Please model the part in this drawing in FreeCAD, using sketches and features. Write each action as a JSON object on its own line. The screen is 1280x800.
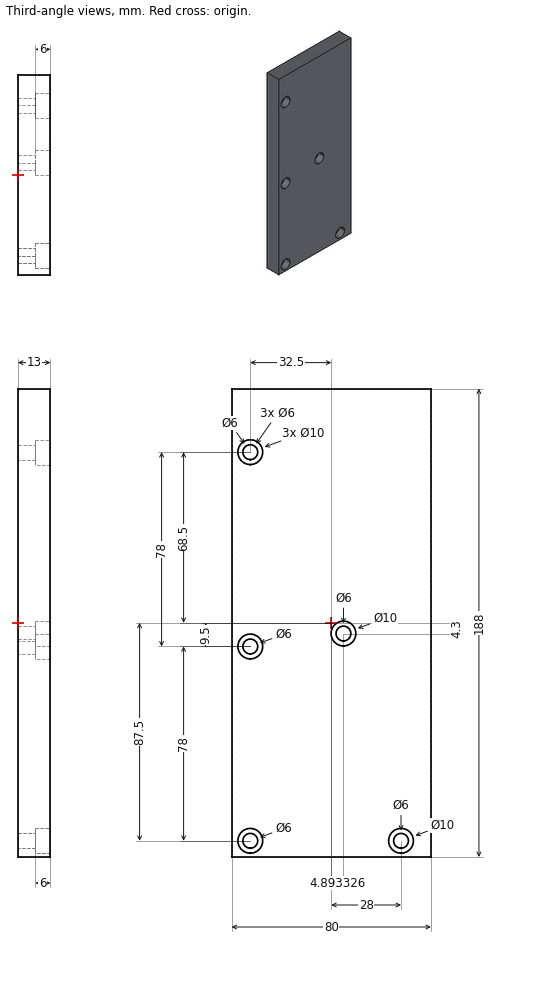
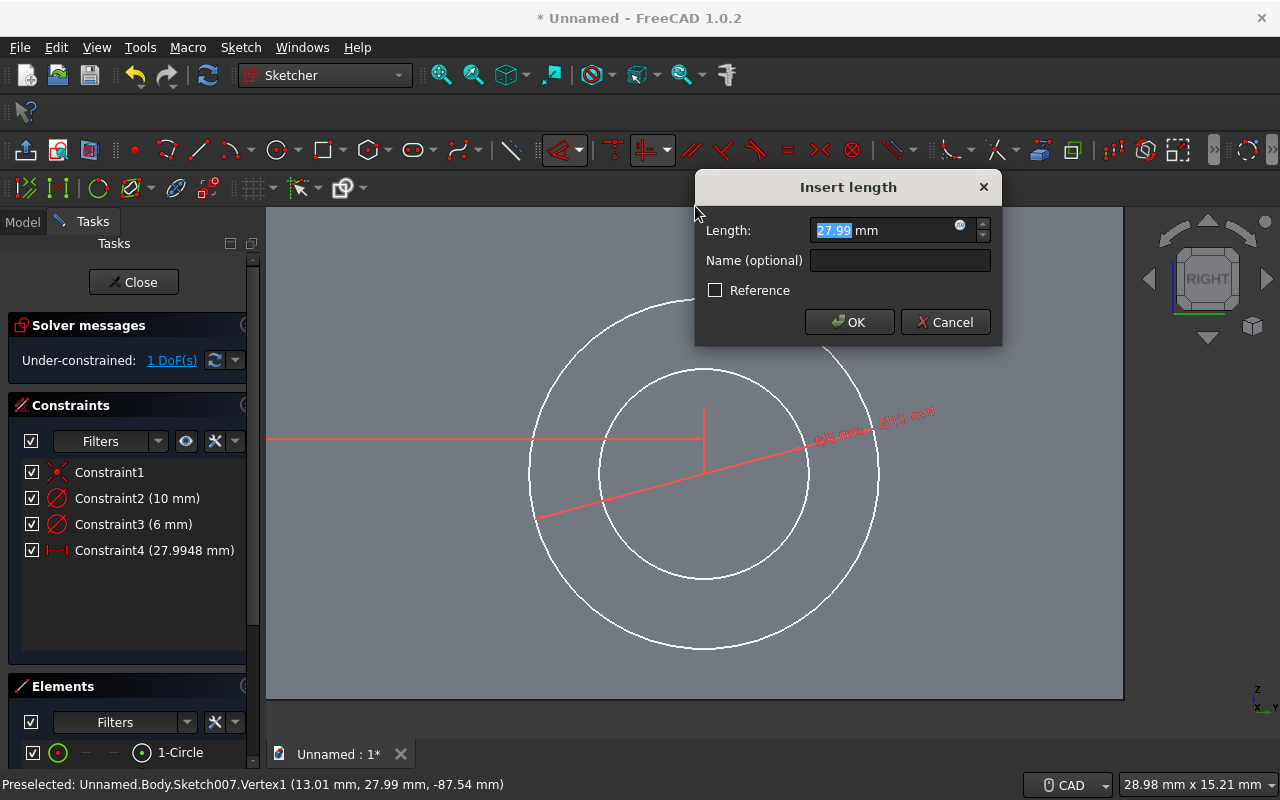
{"action": "type", "text": "28"}
{"action": "key", "text": "Return"}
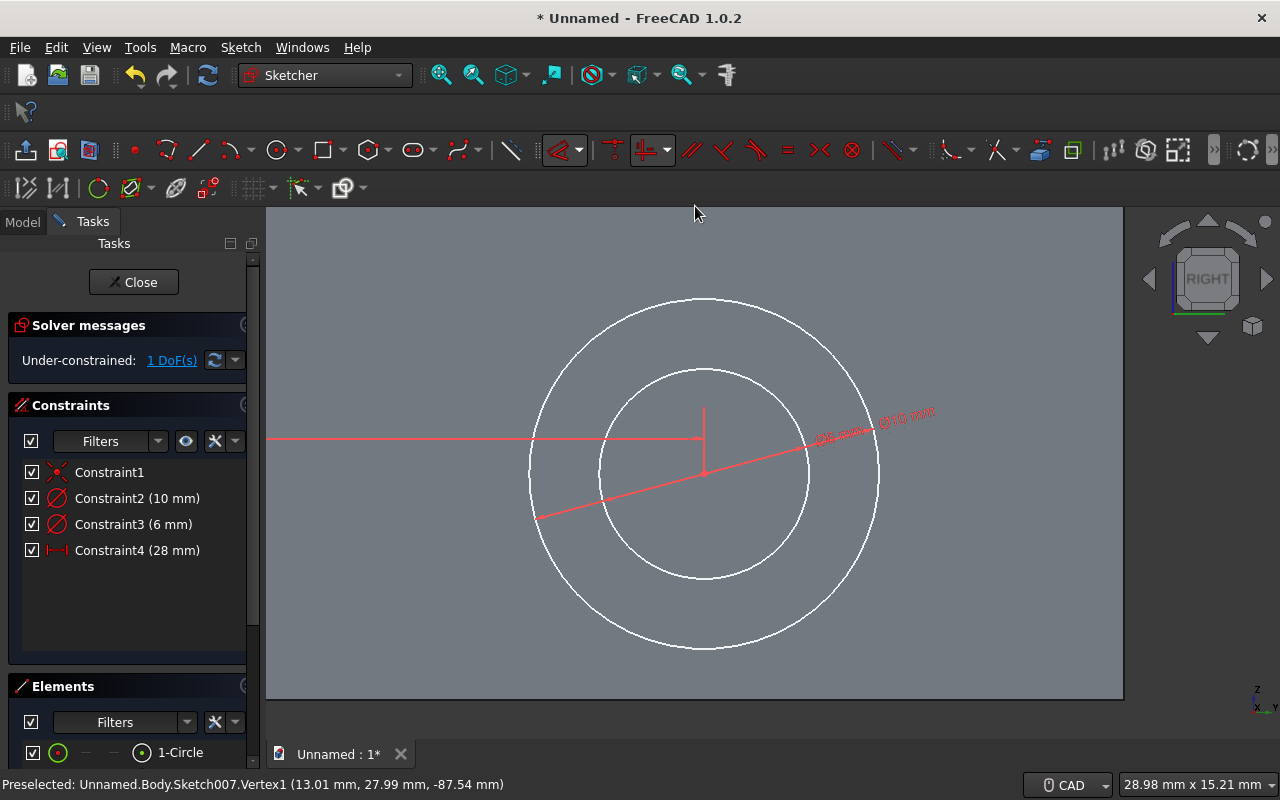
{"action": "left_click", "coordinate": [704, 474]}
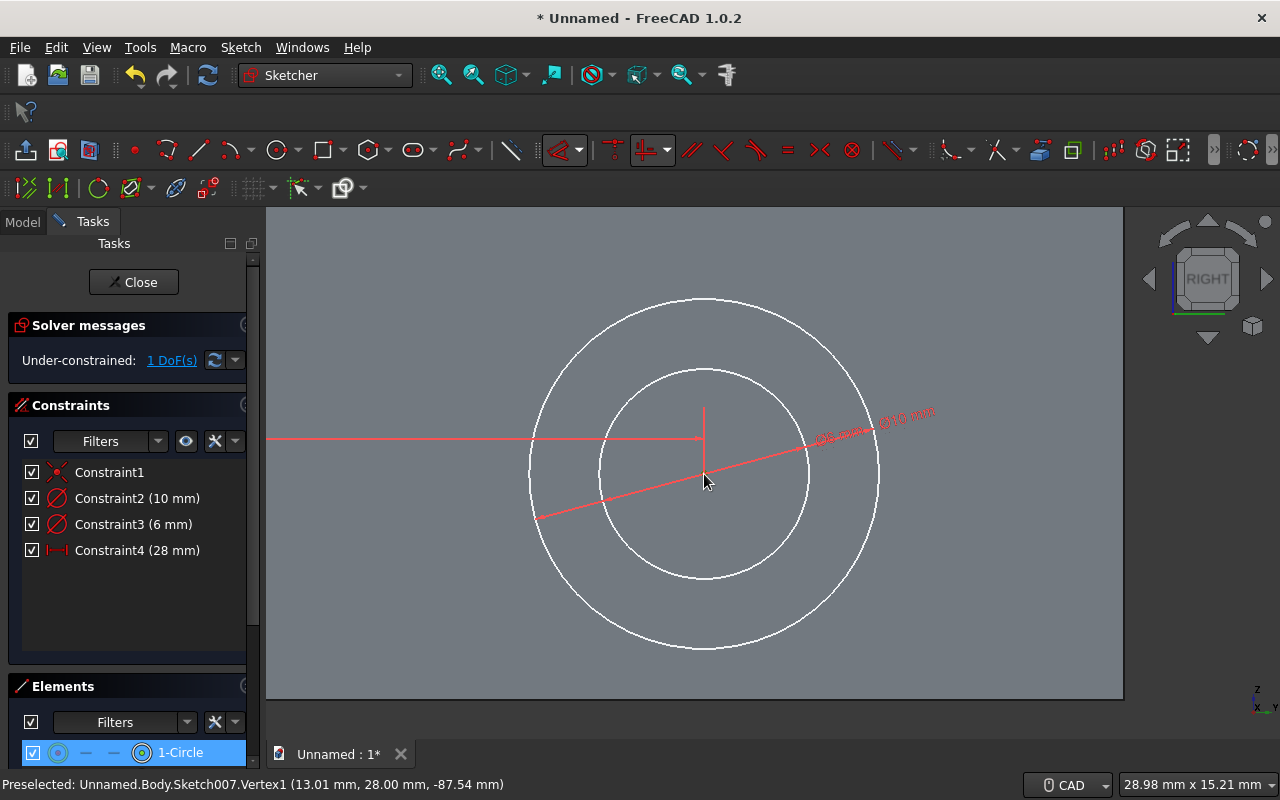
{"action": "key", "text": "i"}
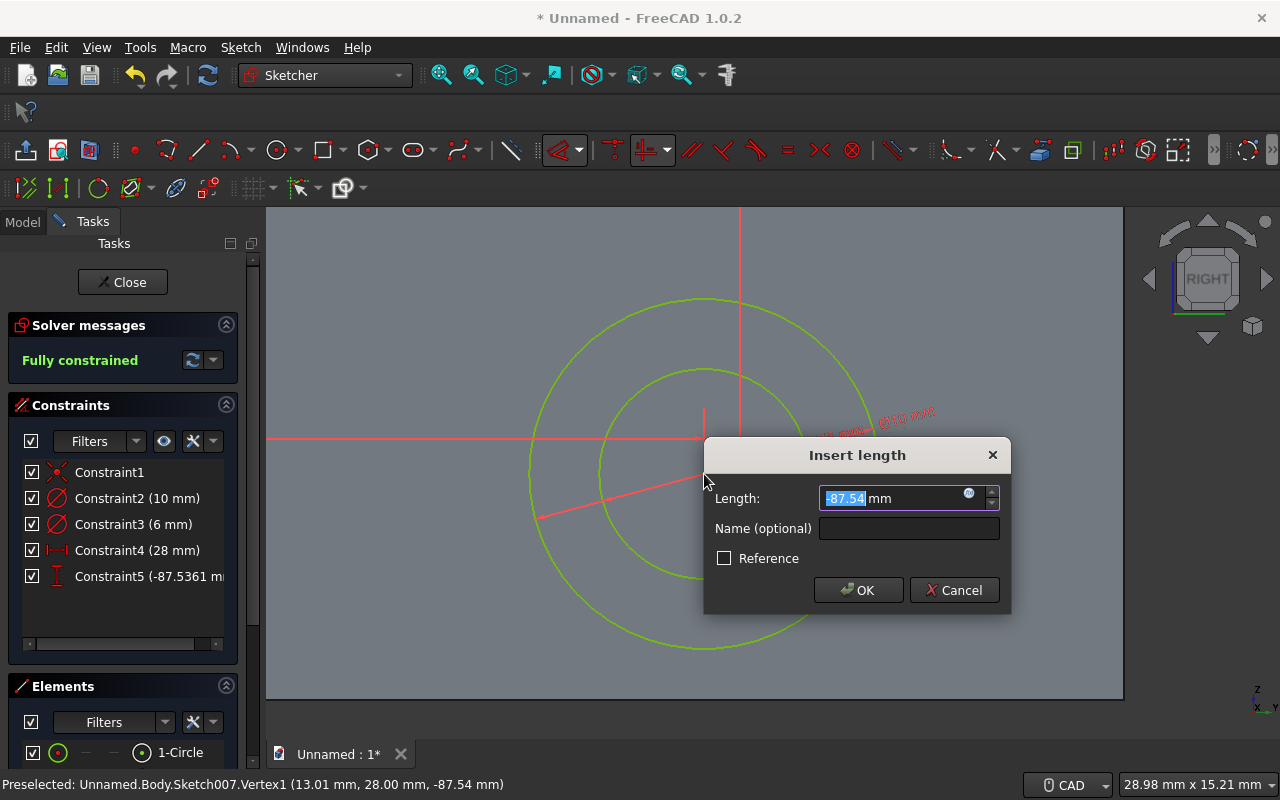
{"action": "type", "text": "-87.5"}
{"action": "key", "text": "Return"}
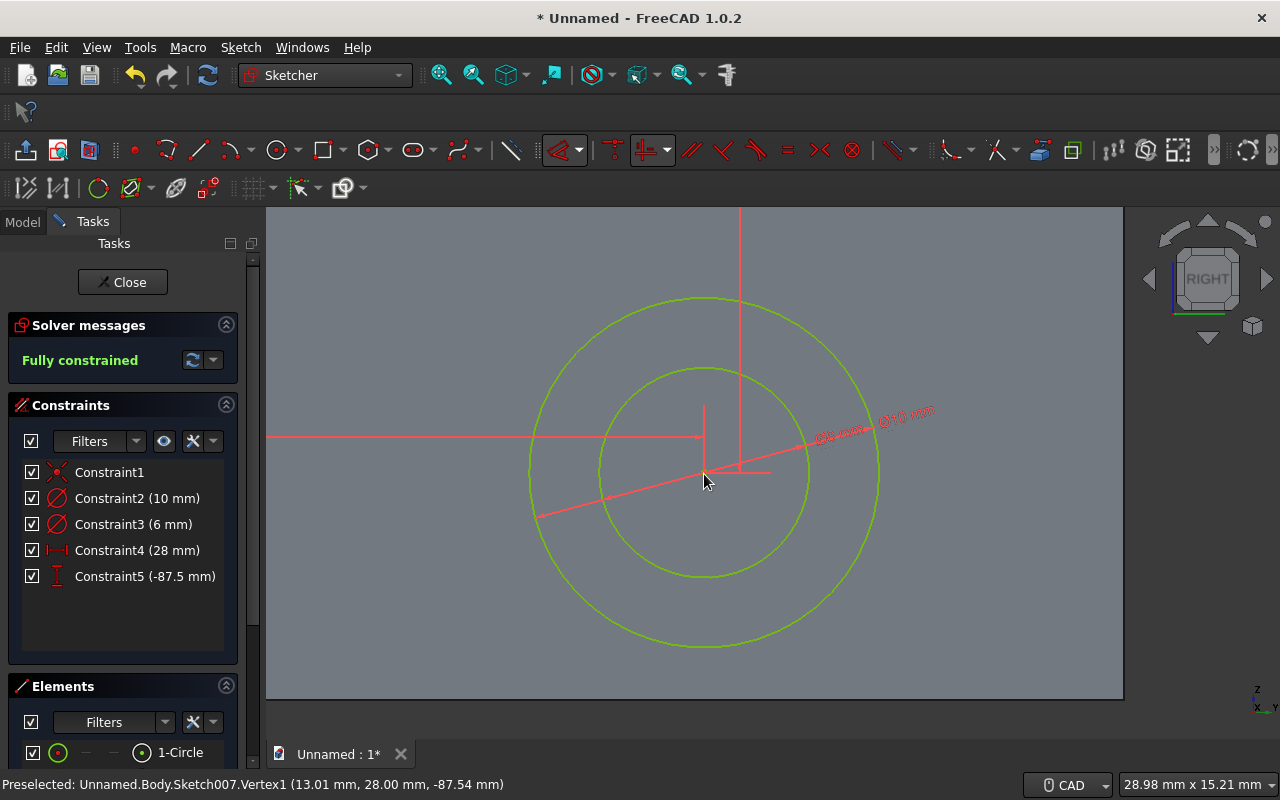
{"action": "left_click", "coordinate": [123, 282]}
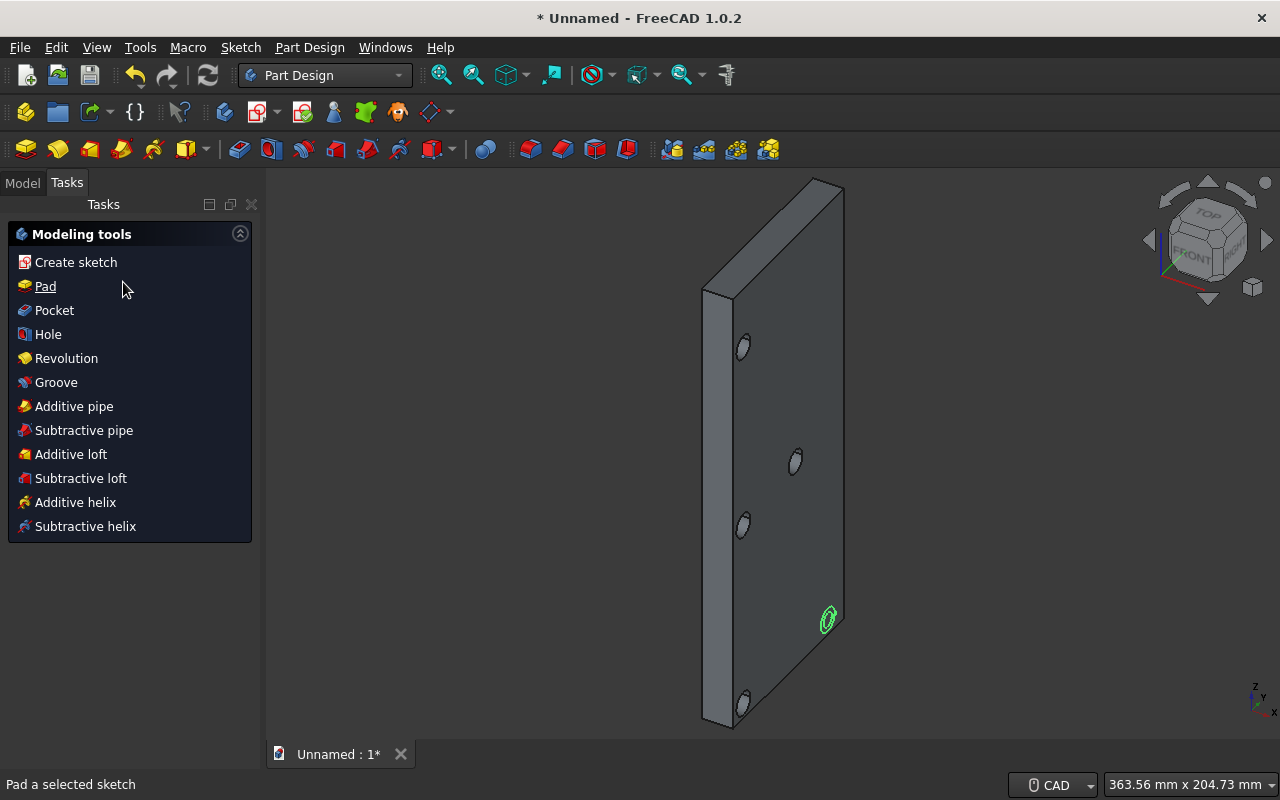
{"action": "left_click", "coordinate": [240, 150]}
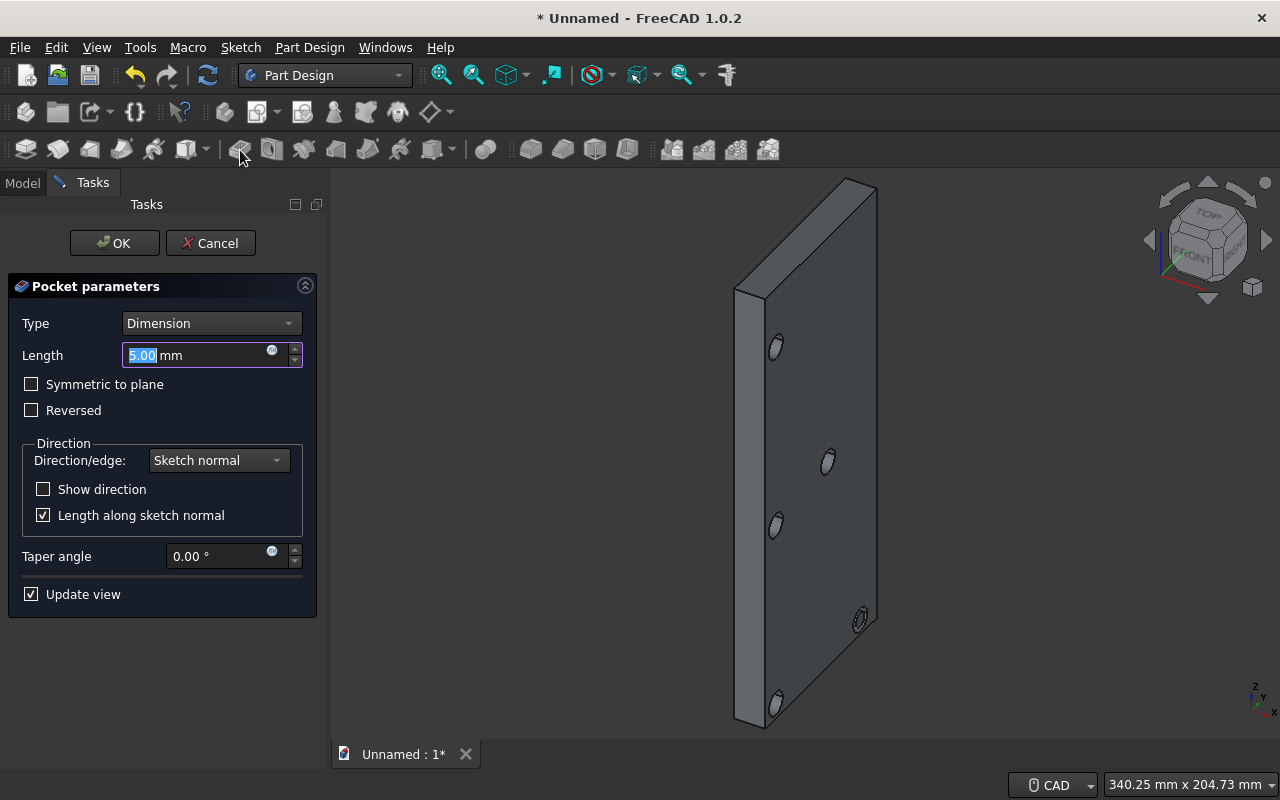
{"action": "type", "text": "6"}
{"action": "key", "text": "Tab"}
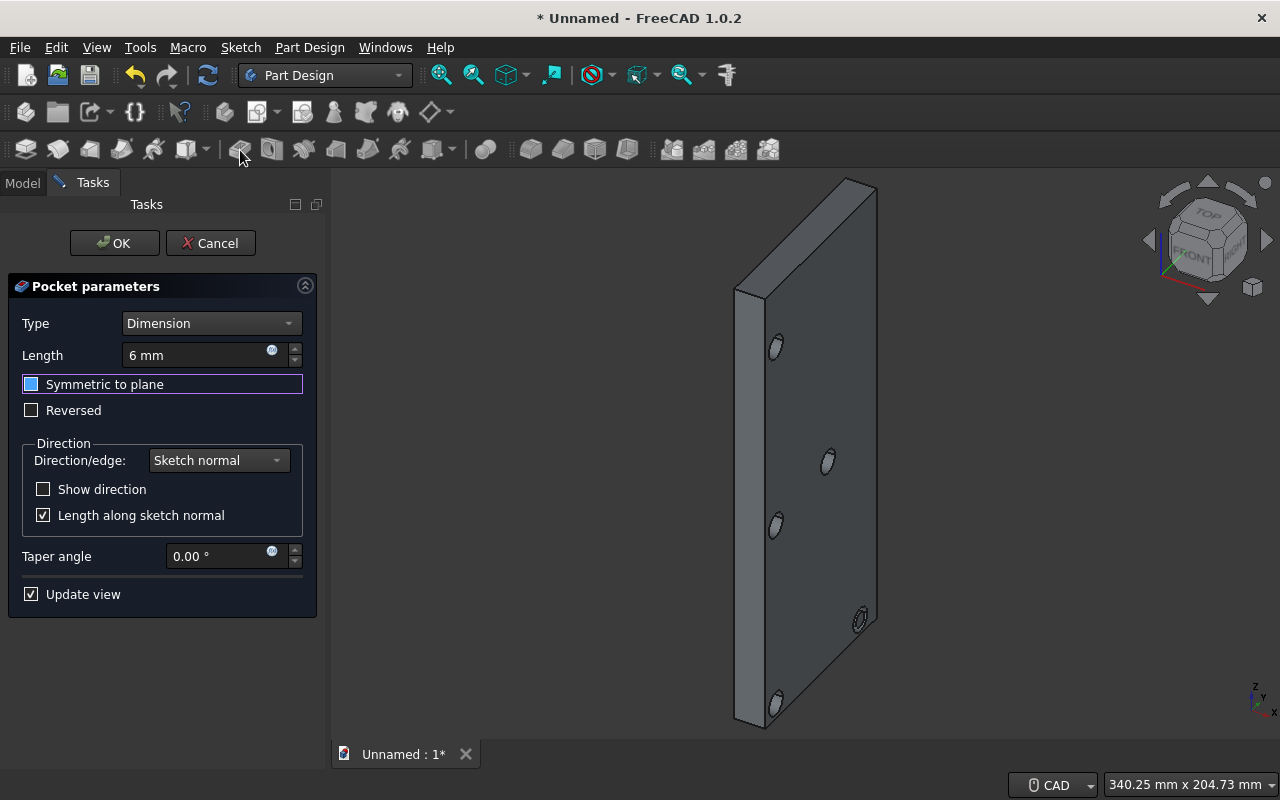
{"action": "left_click", "coordinate": [115, 243]}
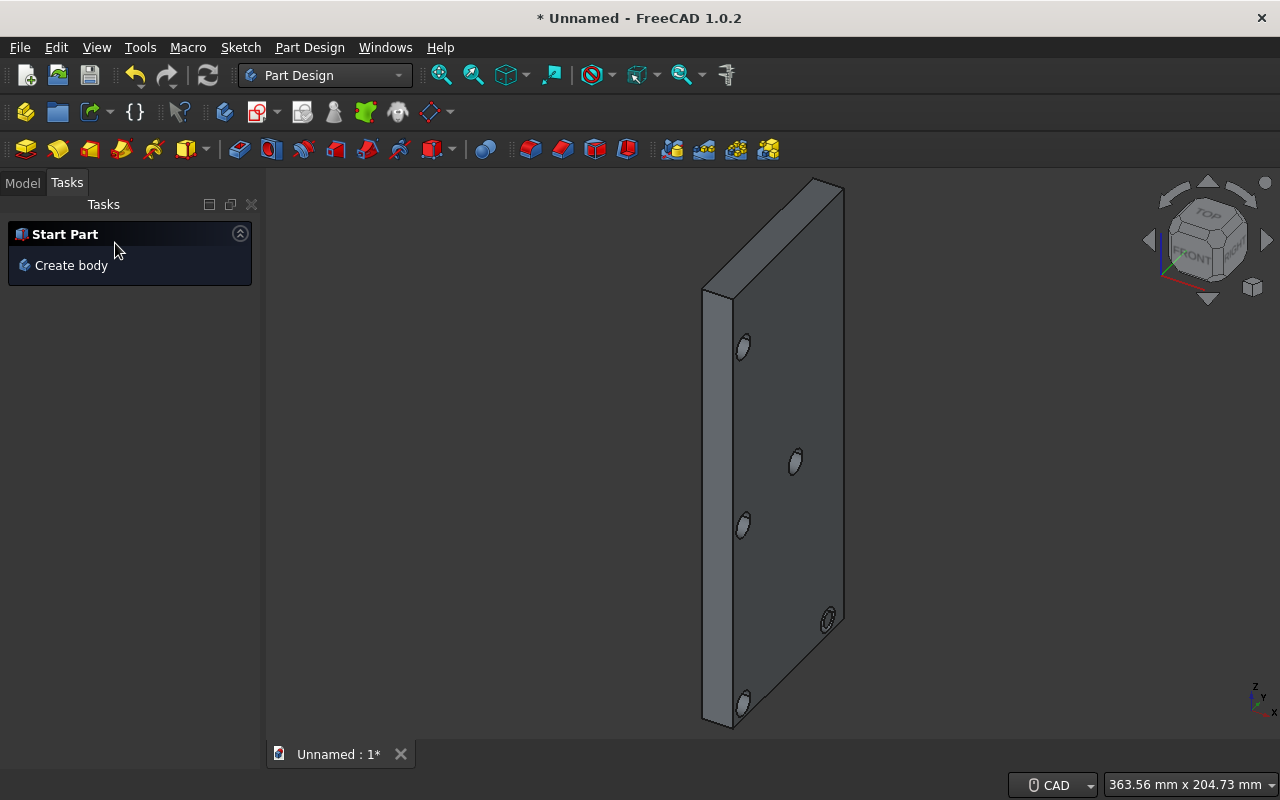
{"action": "left_click", "coordinate": [789, 580]}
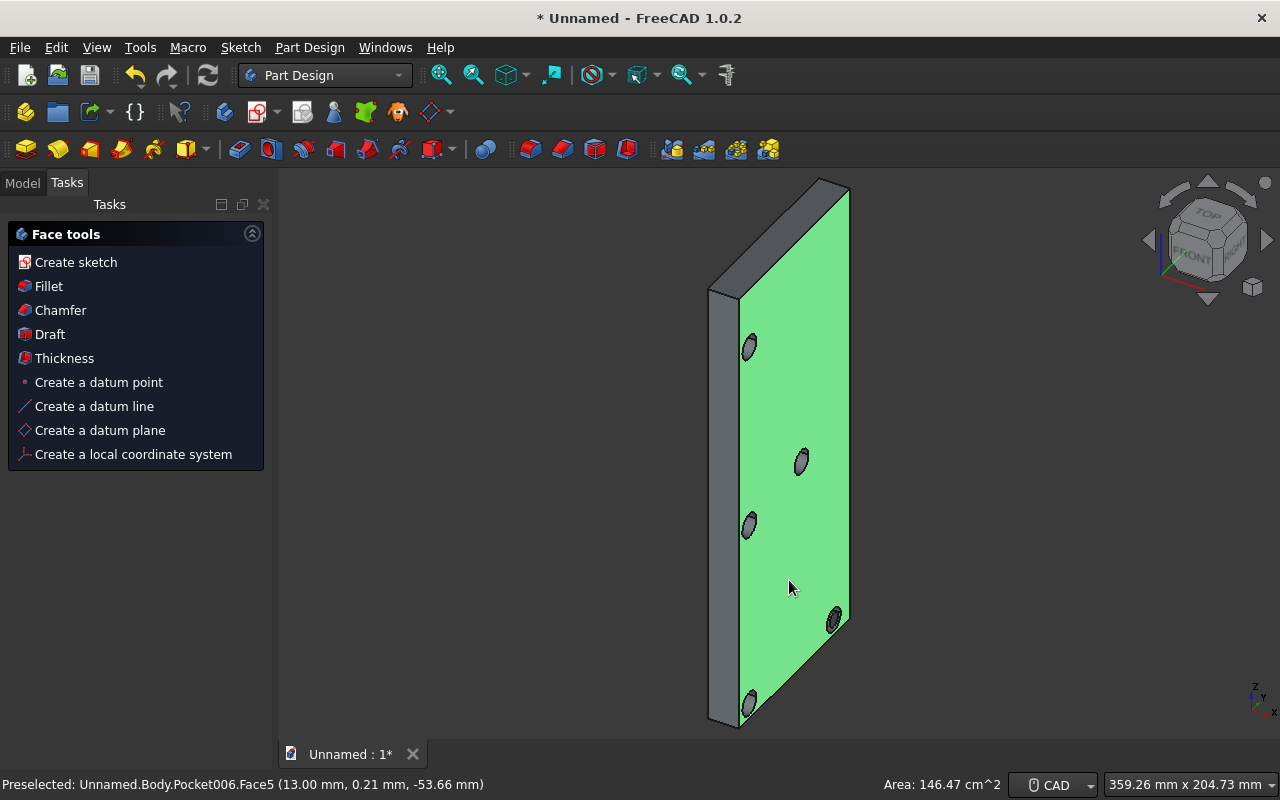
{"action": "left_click", "coordinate": [258, 112]}